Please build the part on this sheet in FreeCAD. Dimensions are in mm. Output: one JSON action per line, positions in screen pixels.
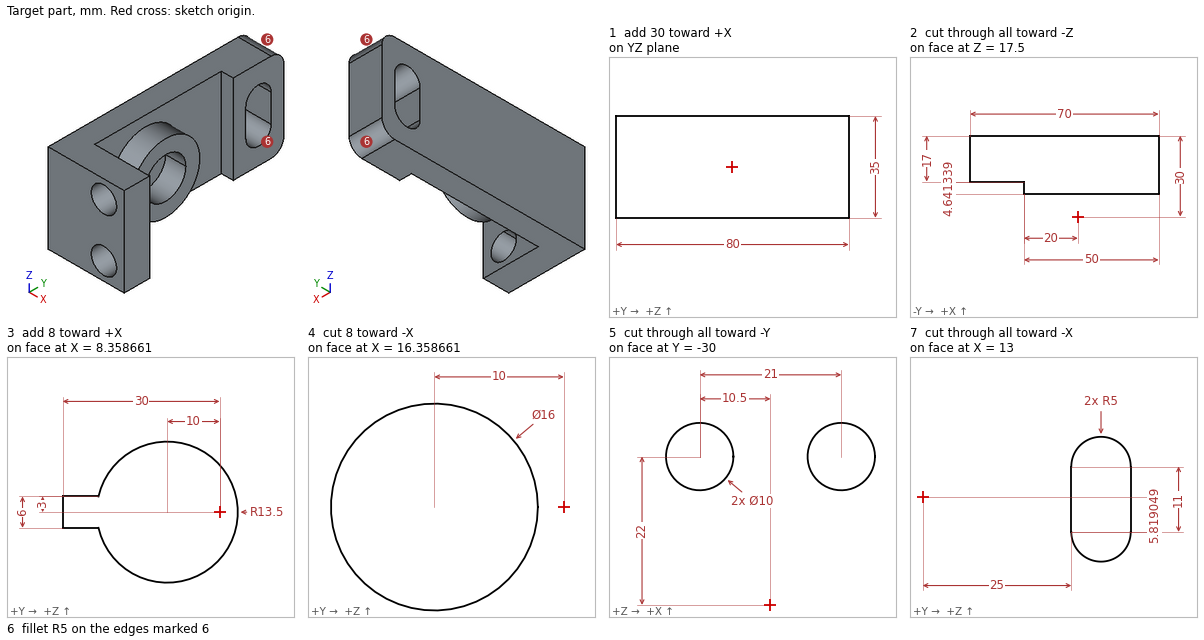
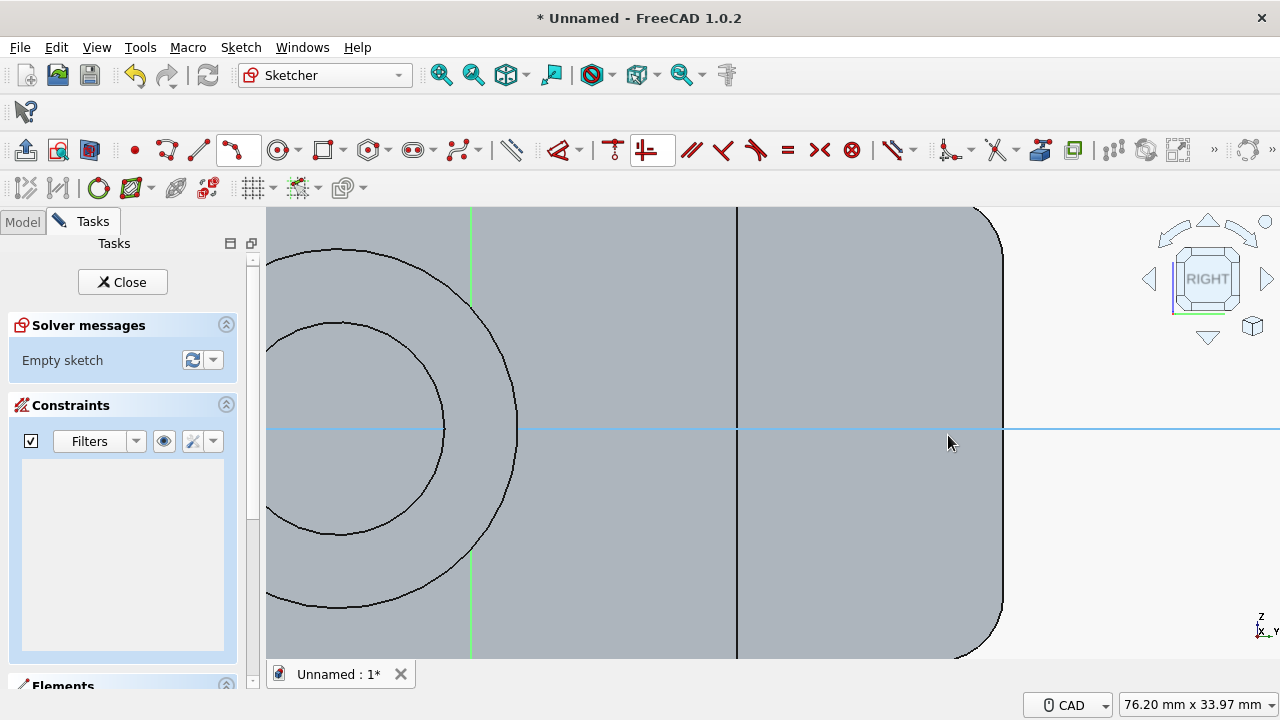
{"action": "left_click", "coordinate": [414, 150]}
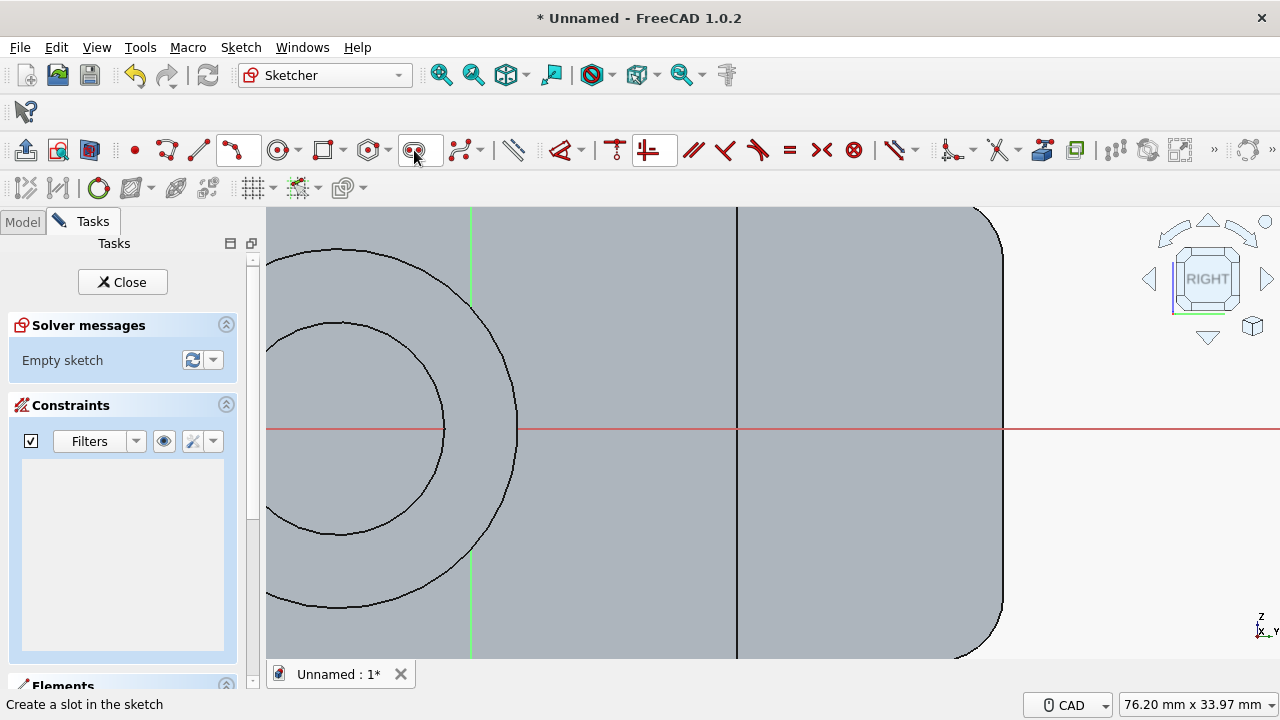
{"action": "left_click", "coordinate": [870, 506]}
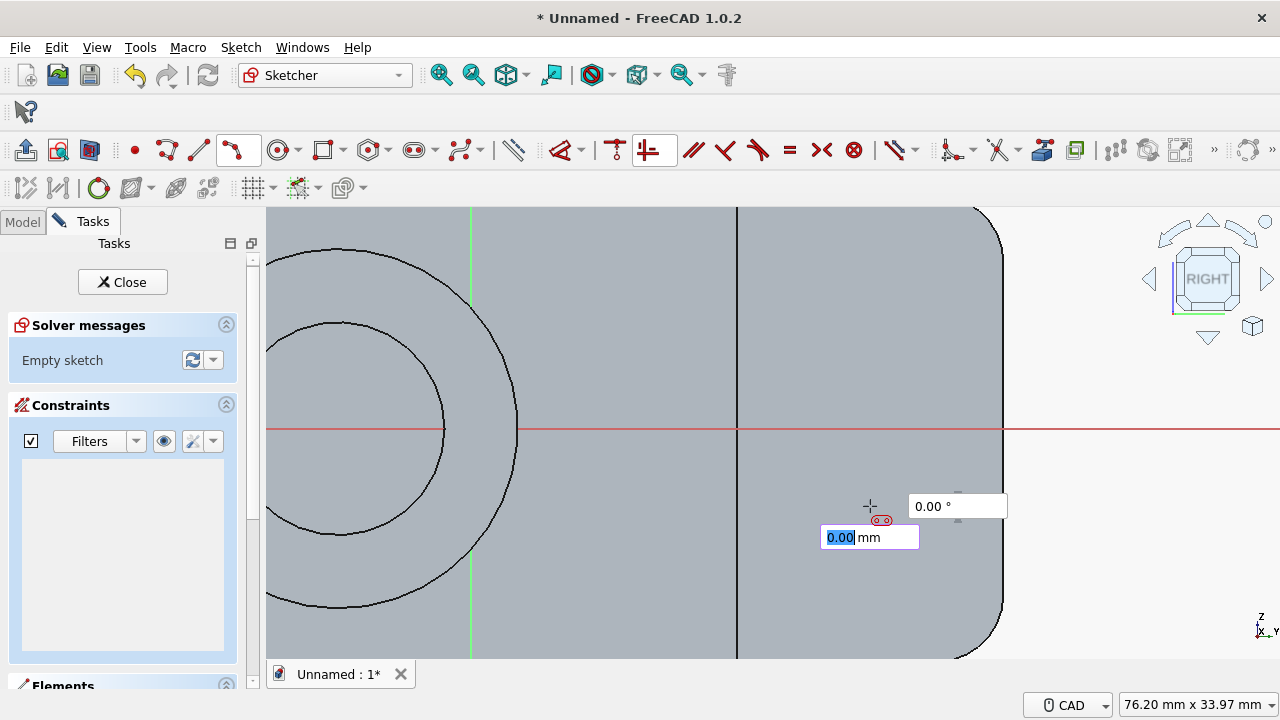
{"action": "left_click", "coordinate": [870, 360]}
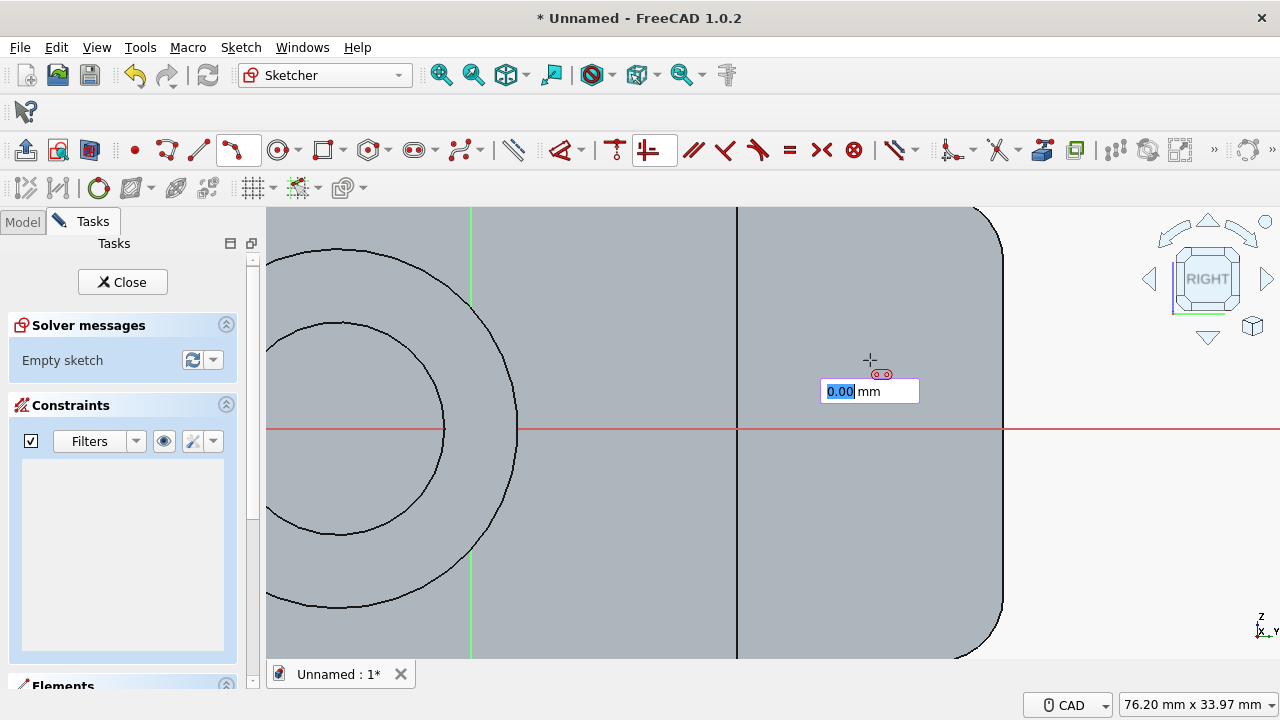
{"action": "left_click", "coordinate": [937, 455]}
{"action": "key", "text": "Escape"}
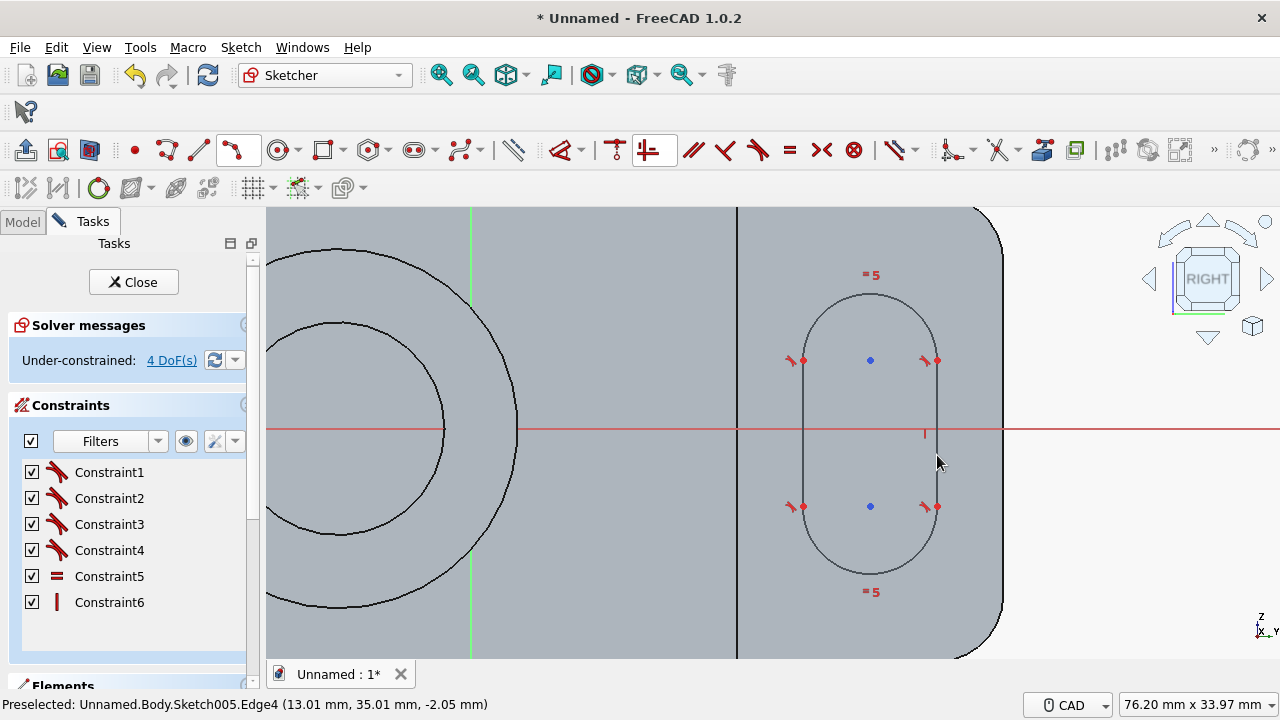
{"action": "left_click", "coordinate": [560, 150]}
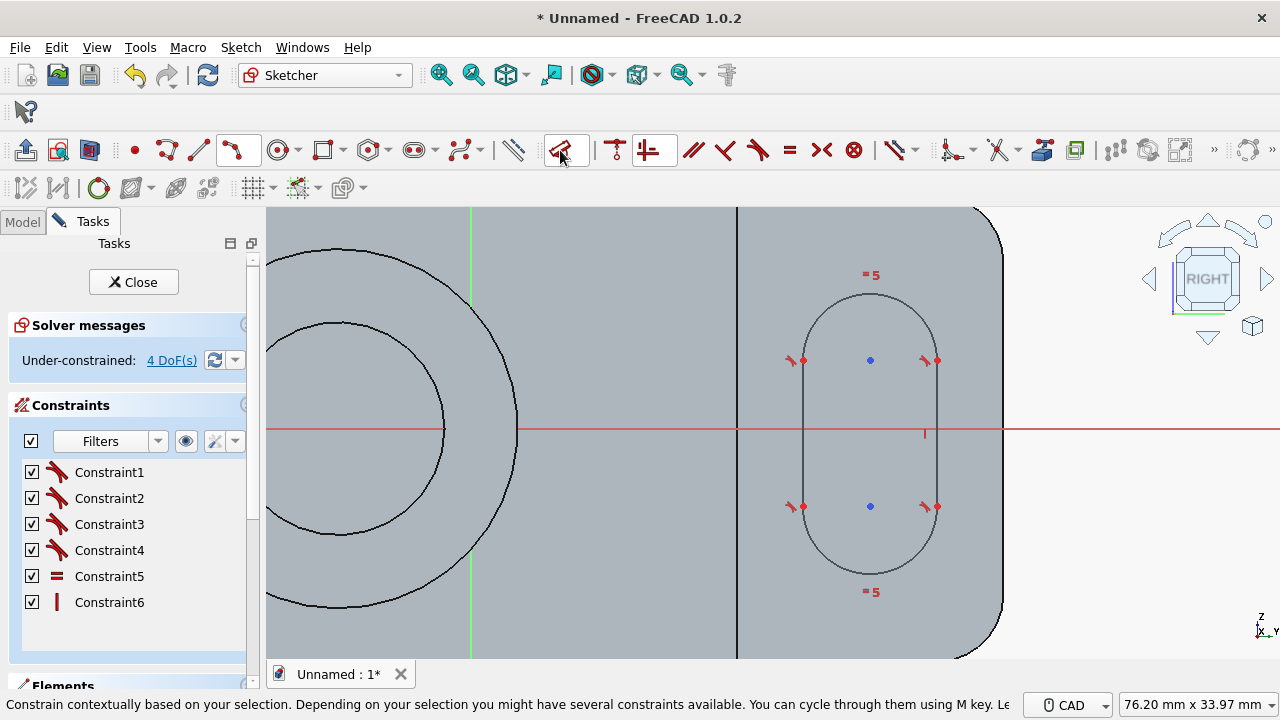
{"action": "left_click", "coordinate": [831, 561]}
{"action": "left_click", "coordinate": [812, 587]}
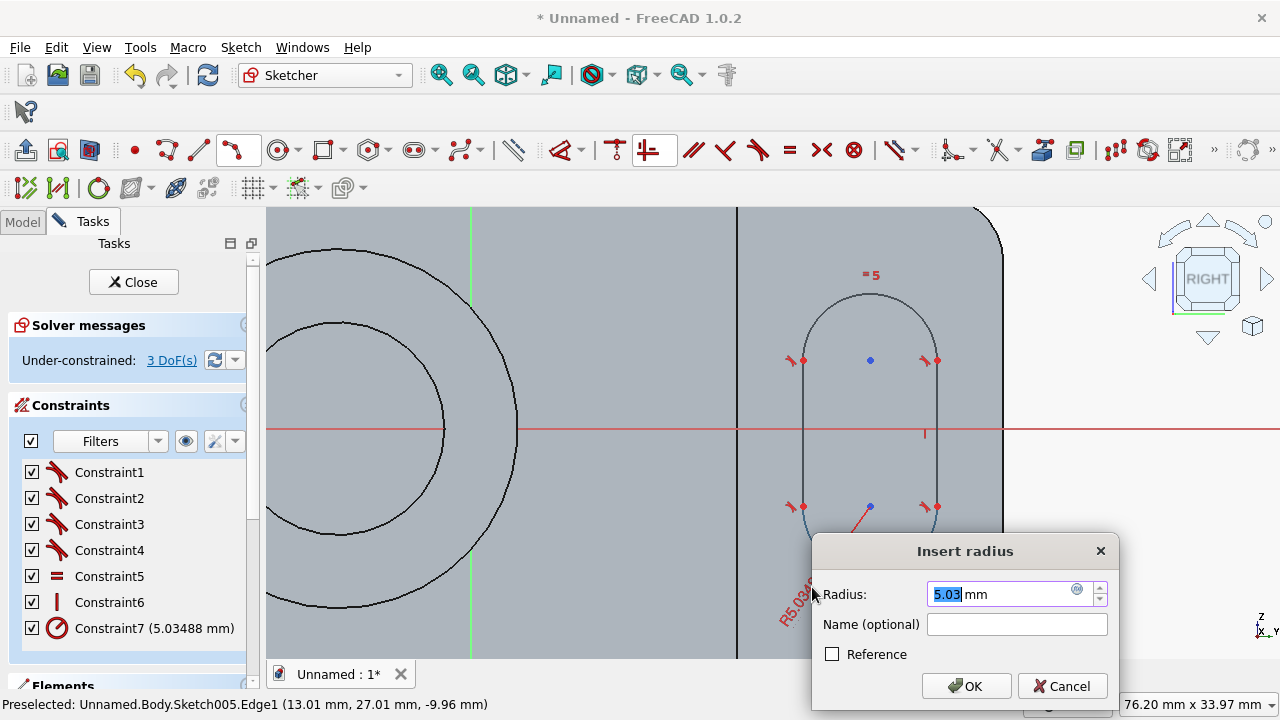
{"action": "type", "text": "5"}
{"action": "key", "text": "Return"}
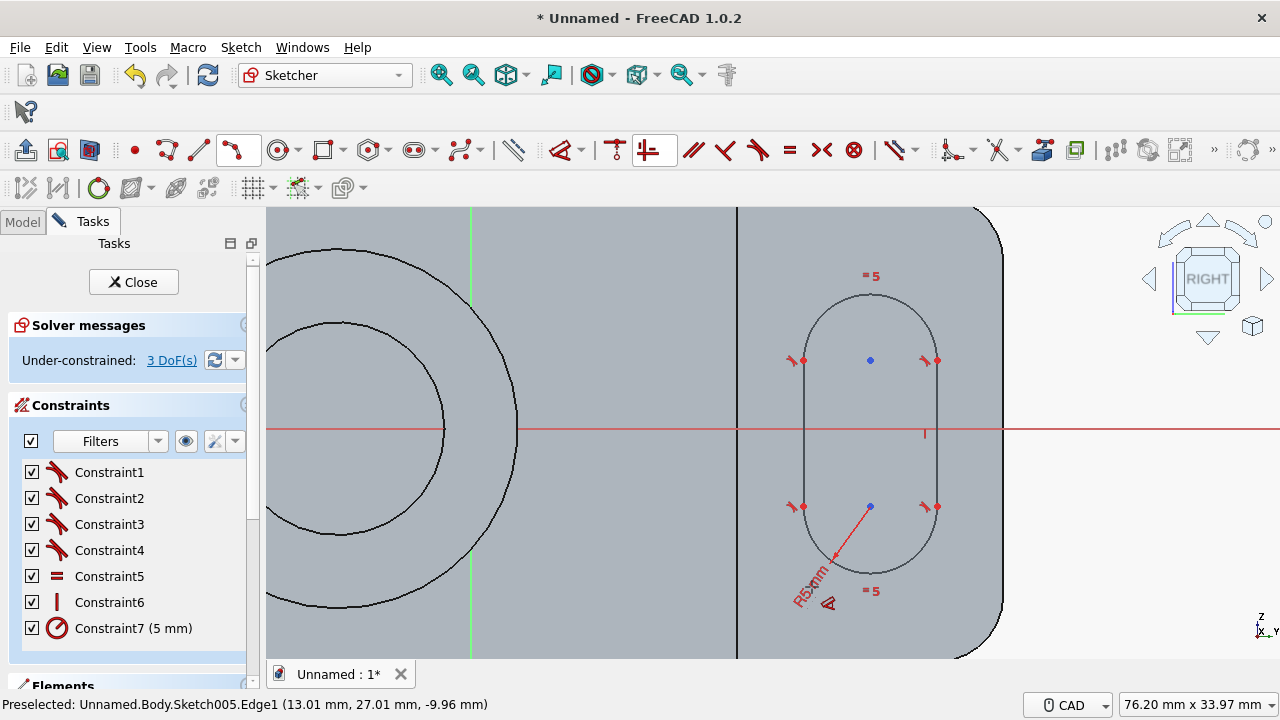
{"action": "left_click", "coordinate": [804, 463]}
{"action": "left_click", "coordinate": [838, 400]}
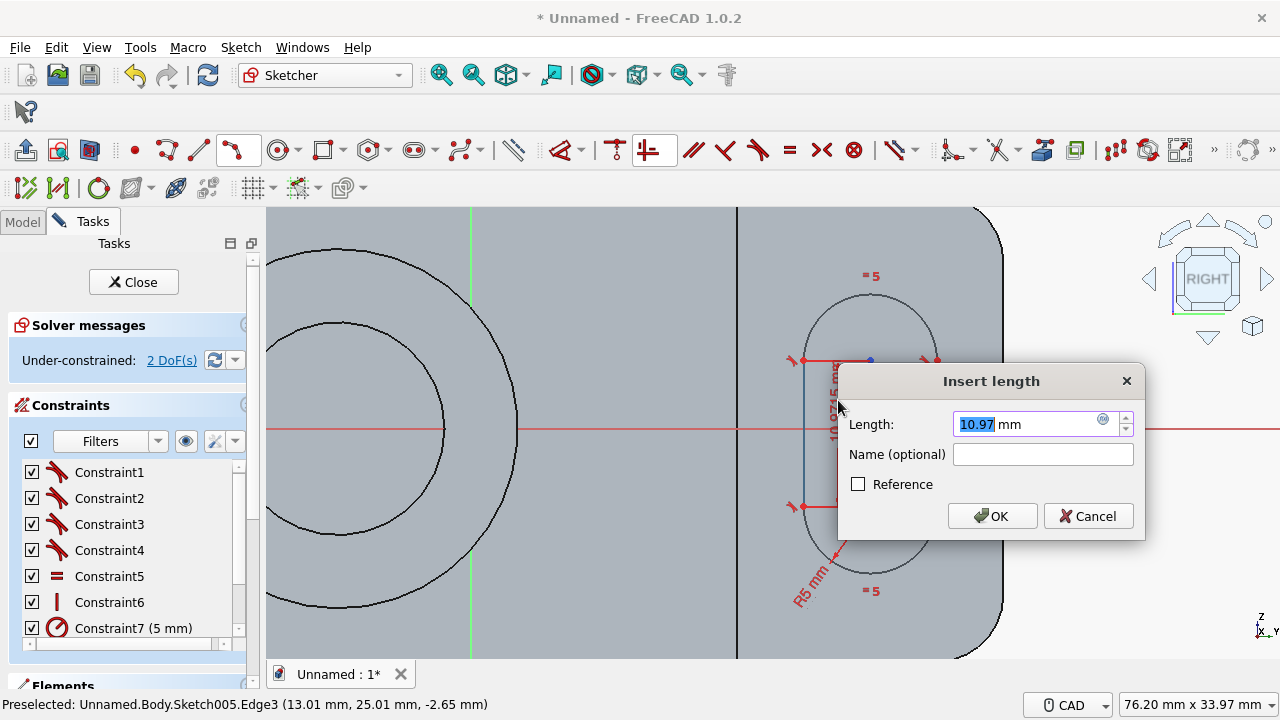
{"action": "type", "text": "11"}
{"action": "key", "text": "Return"}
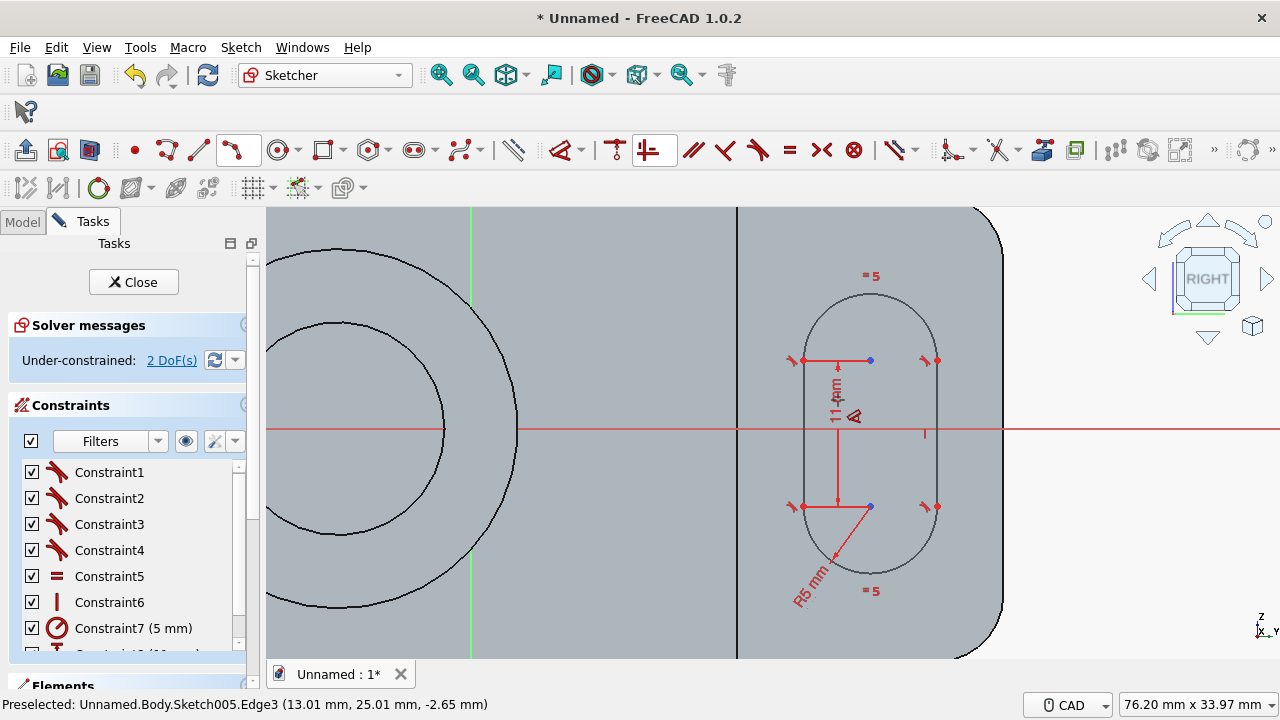
{"action": "left_click", "coordinate": [804, 507]}
{"action": "left_click", "coordinate": [638, 541]}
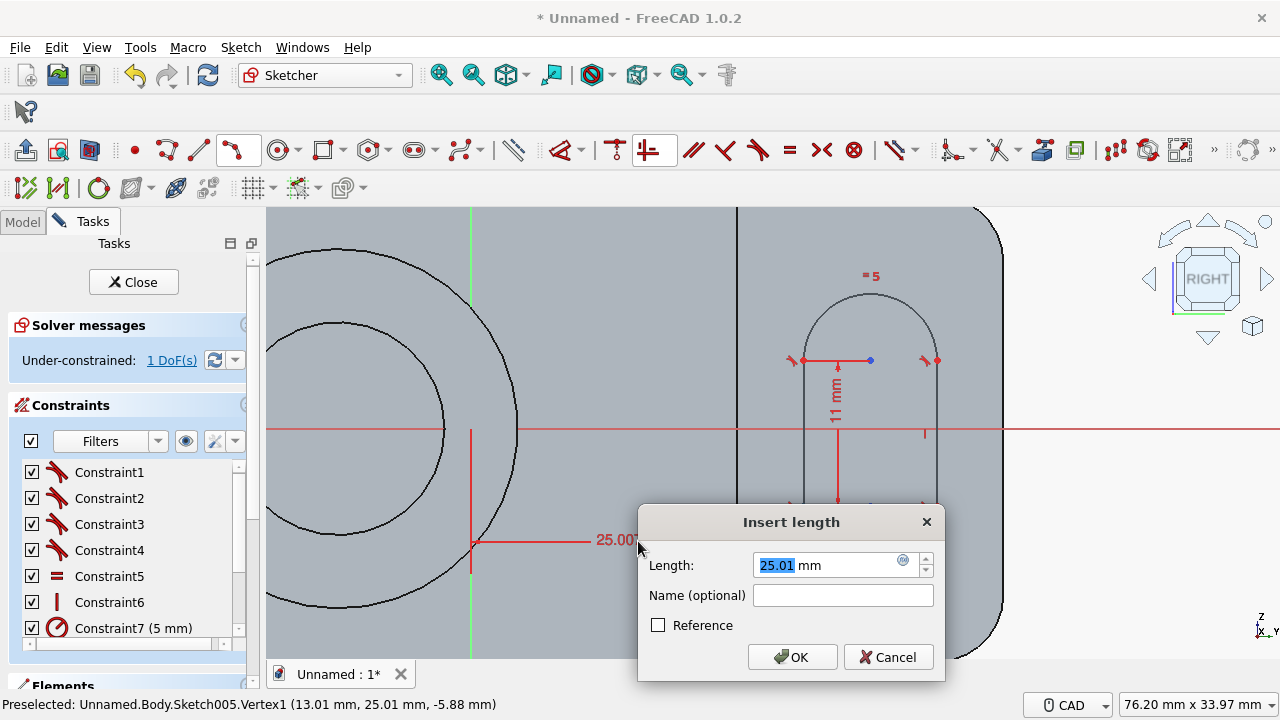
{"action": "type", "text": "25"}
{"action": "key", "text": "Return"}